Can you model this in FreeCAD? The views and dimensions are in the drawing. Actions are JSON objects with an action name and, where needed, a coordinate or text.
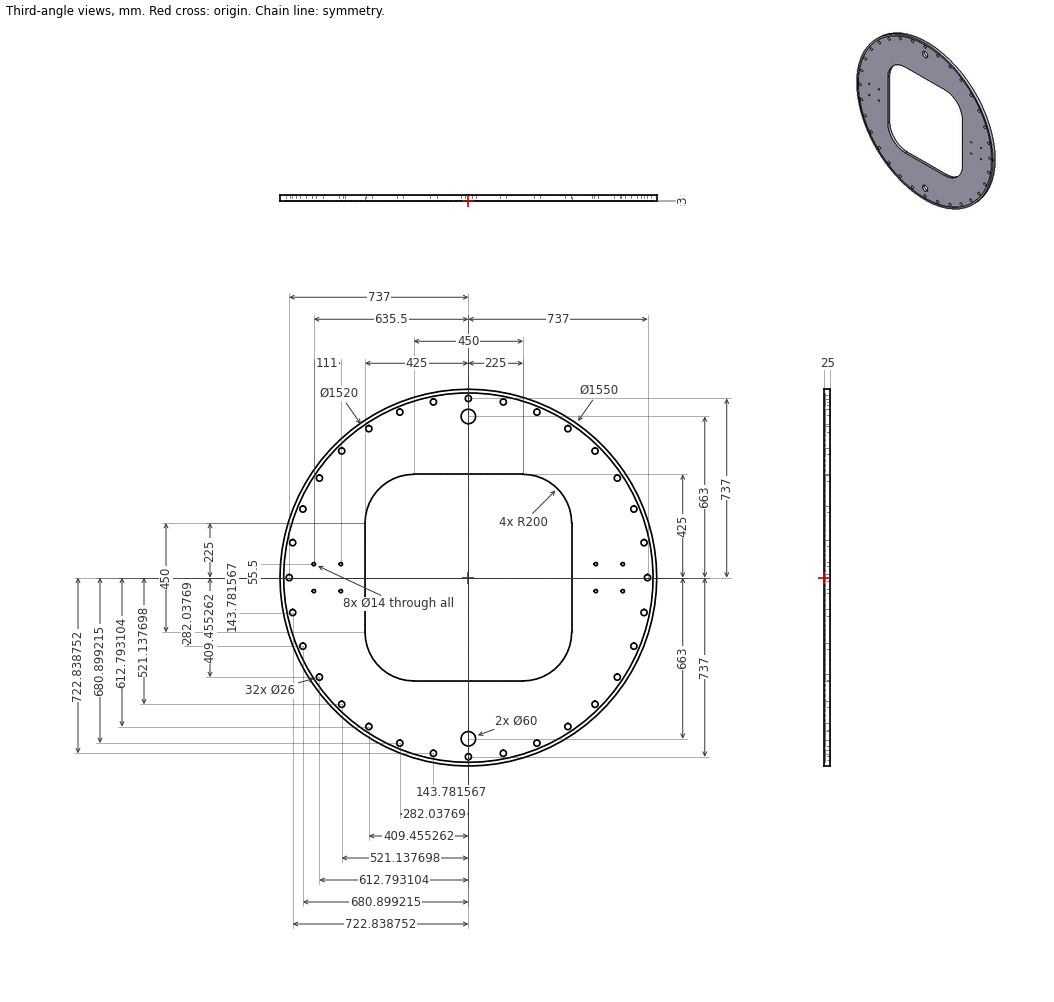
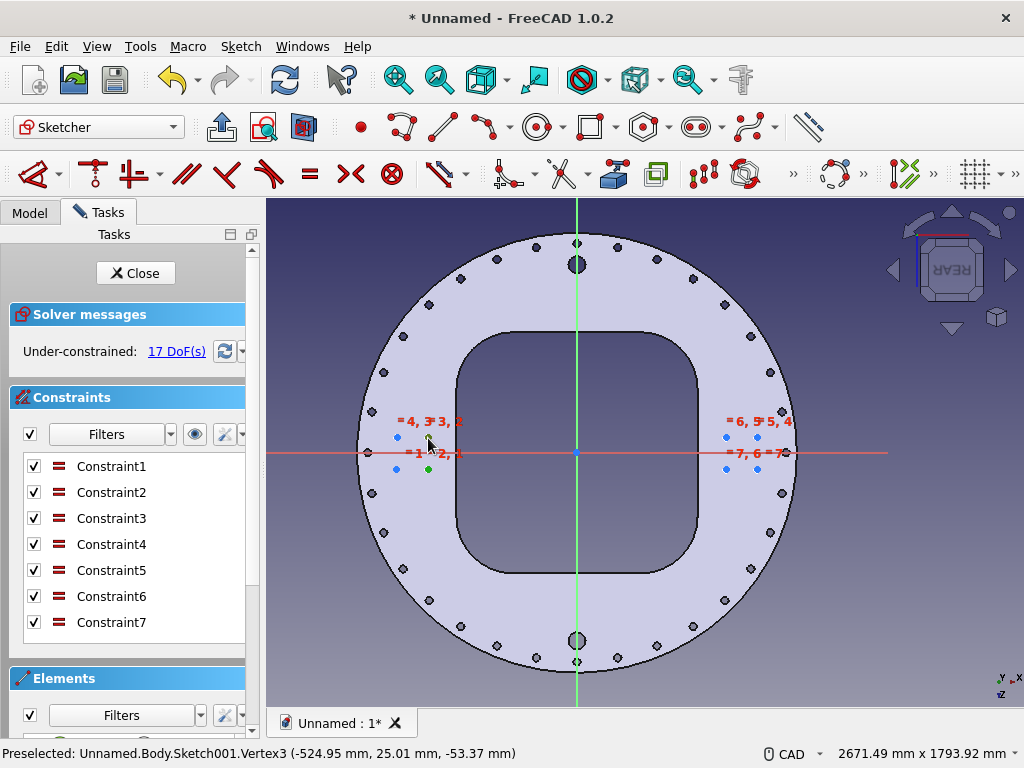
{"action": "left_click", "coordinate": [334, 453]}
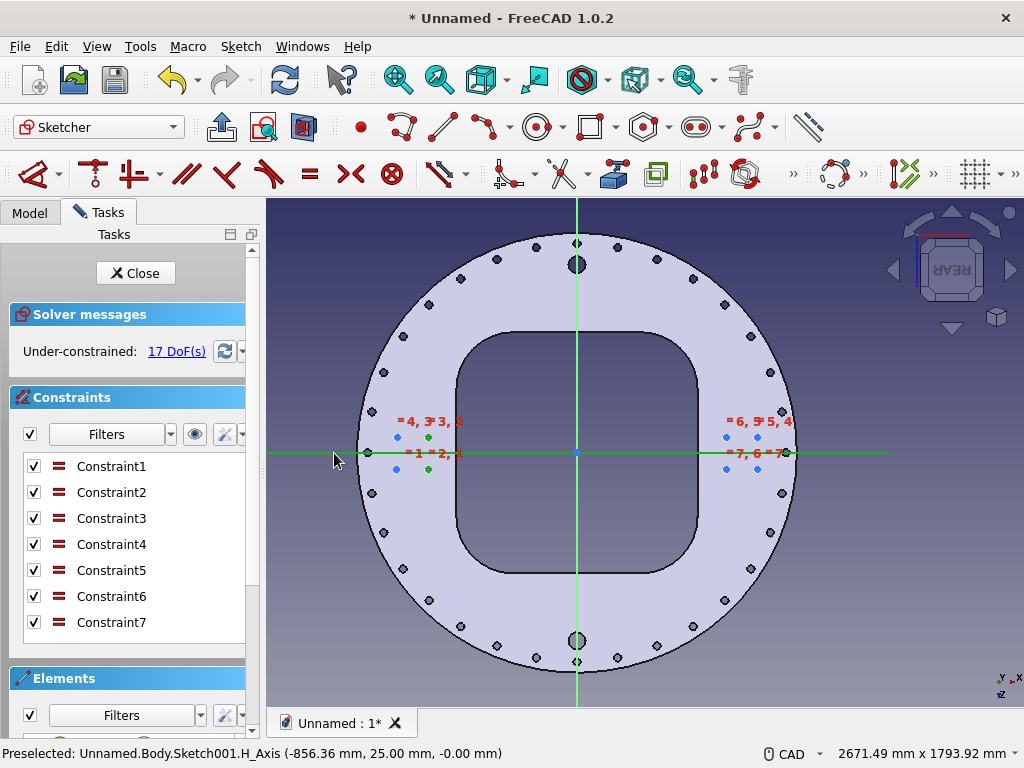
{"action": "left_click", "coordinate": [351, 174]}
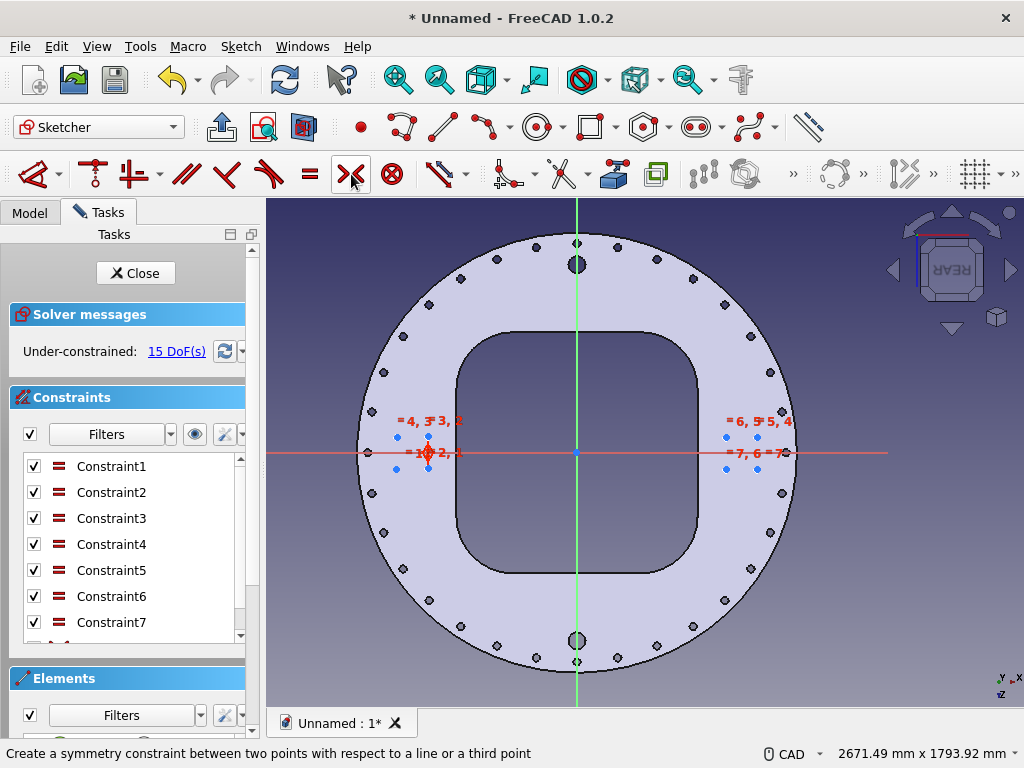
{"action": "left_click", "coordinate": [396, 469]}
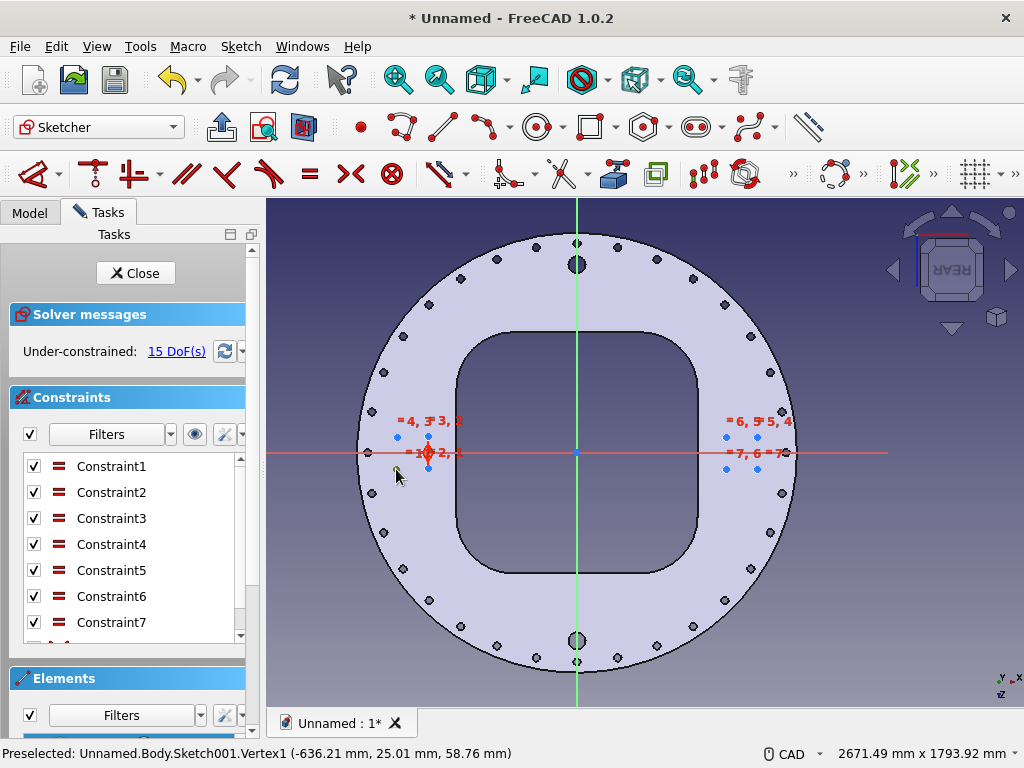
{"action": "left_click", "coordinate": [397, 438]}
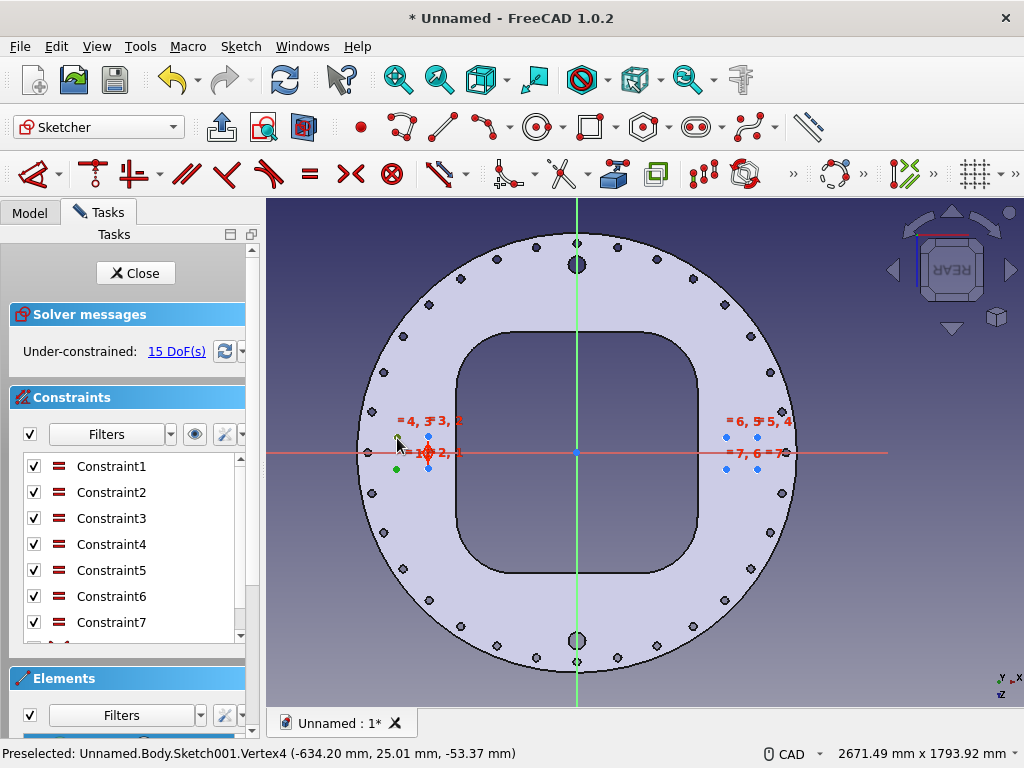
{"action": "left_click", "coordinate": [334, 453]}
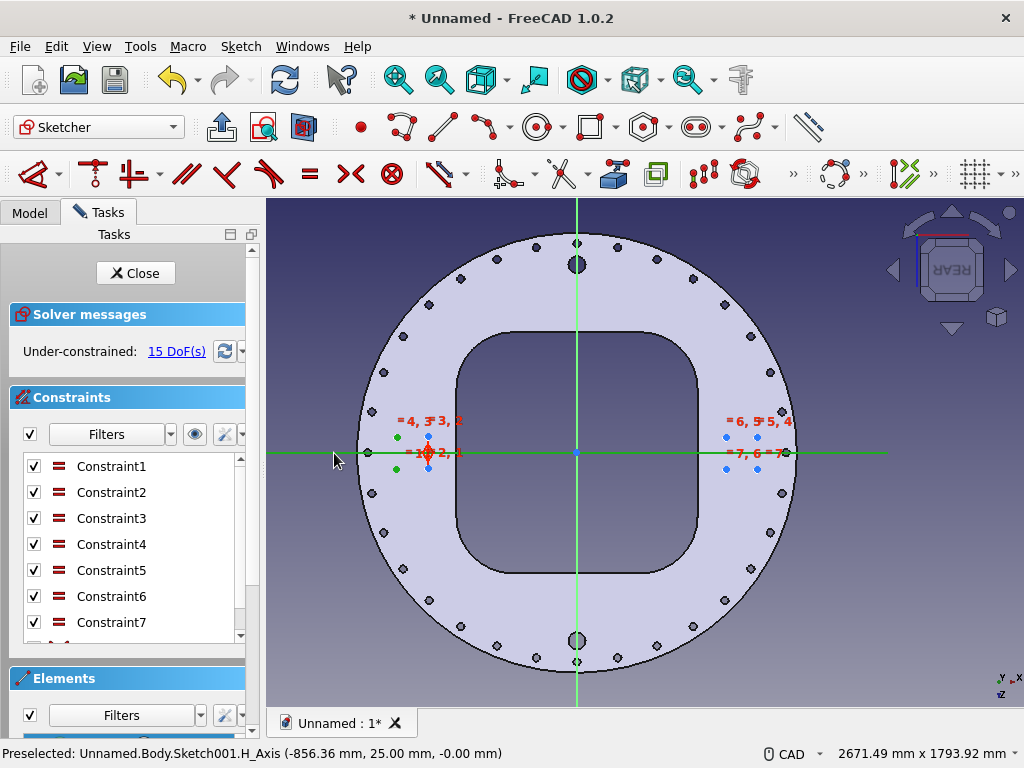
{"action": "left_click", "coordinate": [351, 174]}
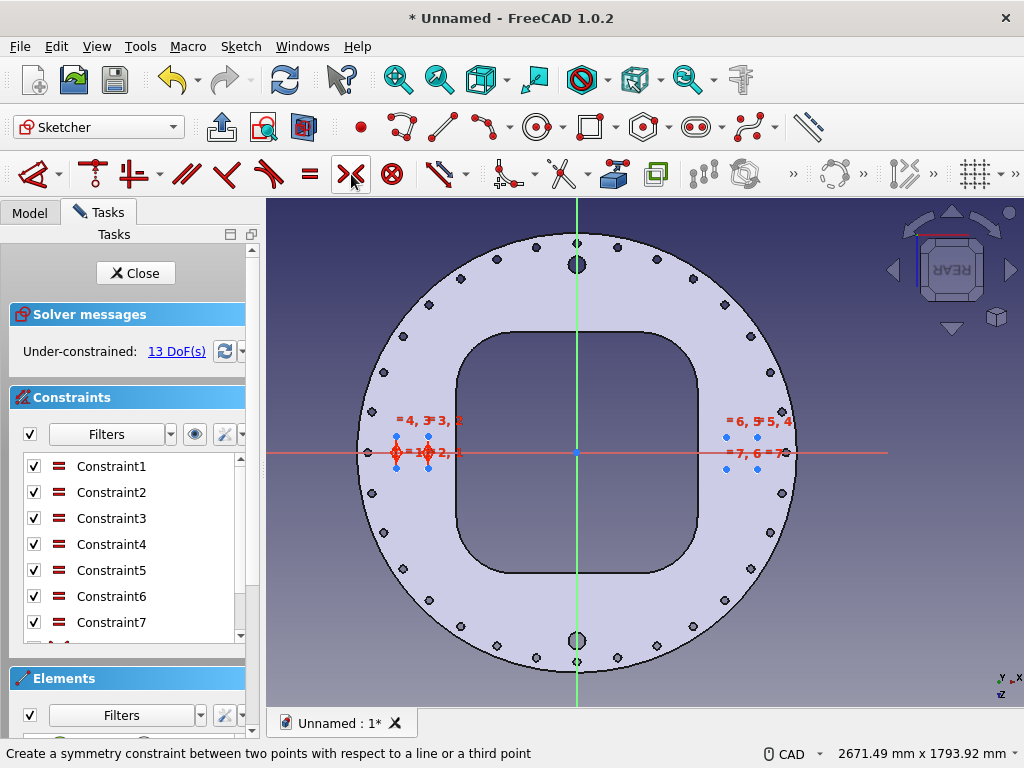
{"action": "left_click", "coordinate": [396, 437]}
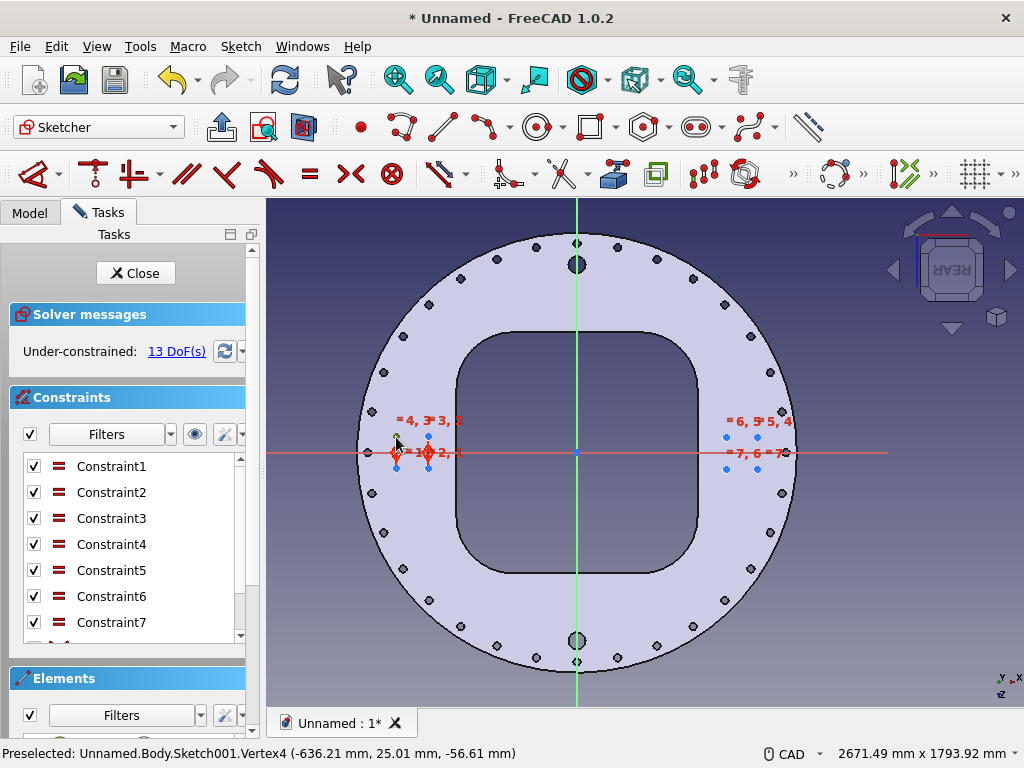
{"action": "left_click", "coordinate": [757, 438]}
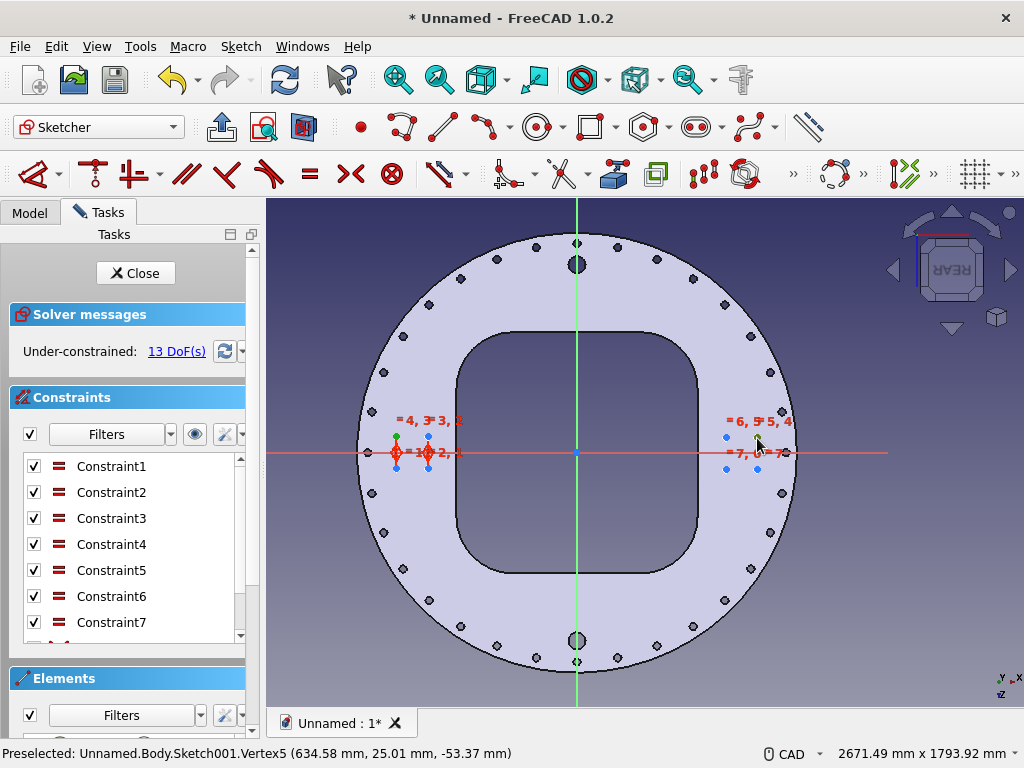
{"action": "left_click", "coordinate": [577, 647]}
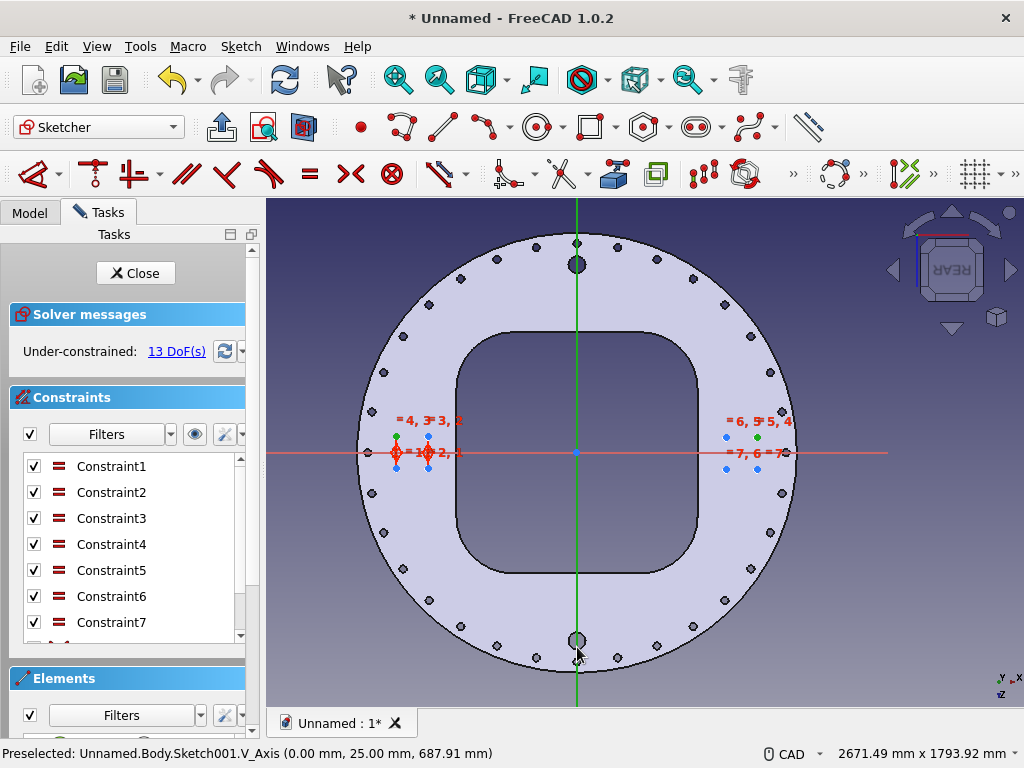
{"action": "left_click", "coordinate": [351, 174]}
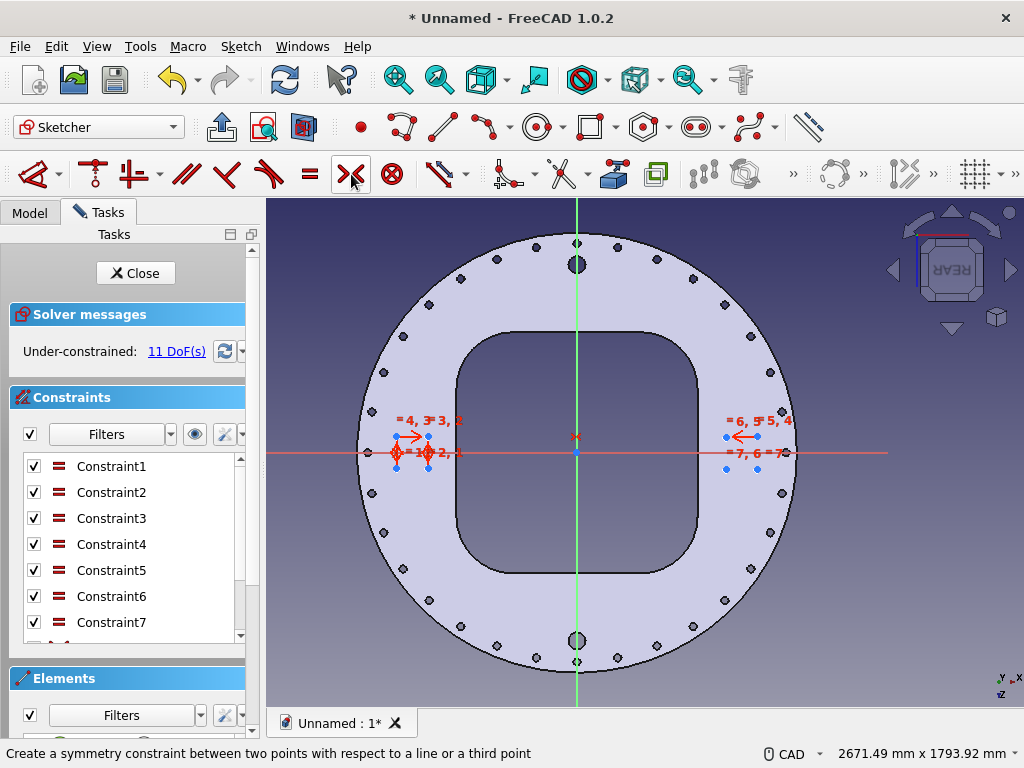
{"action": "left_click", "coordinate": [428, 437]}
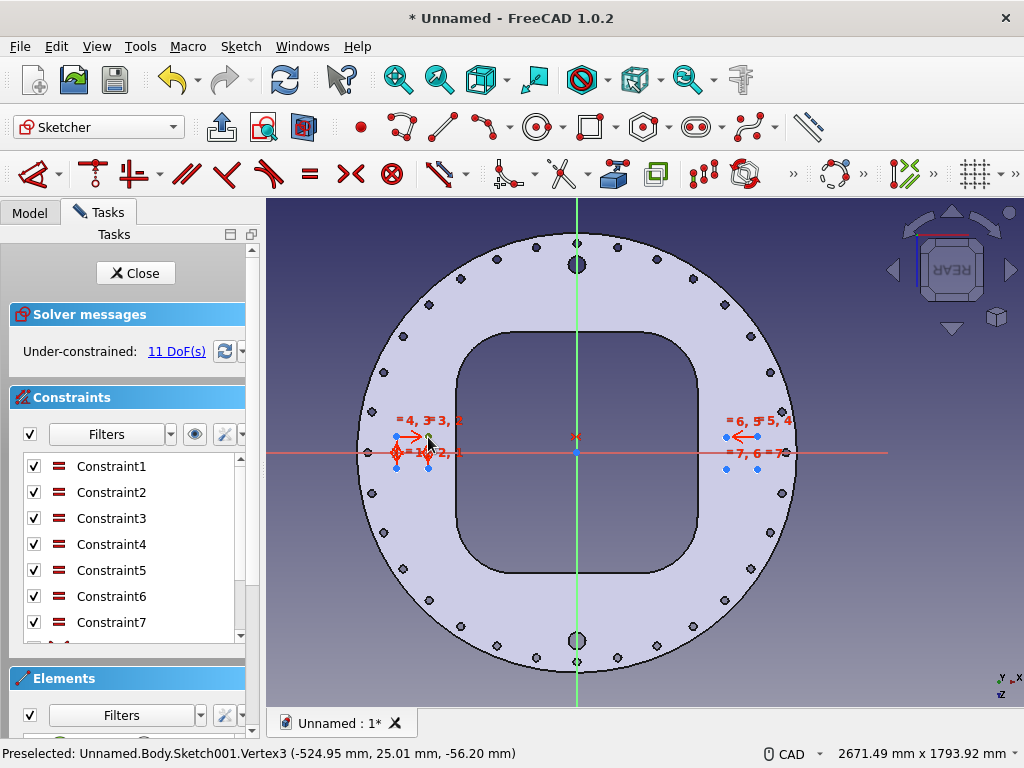
{"action": "left_click", "coordinate": [726, 438]}